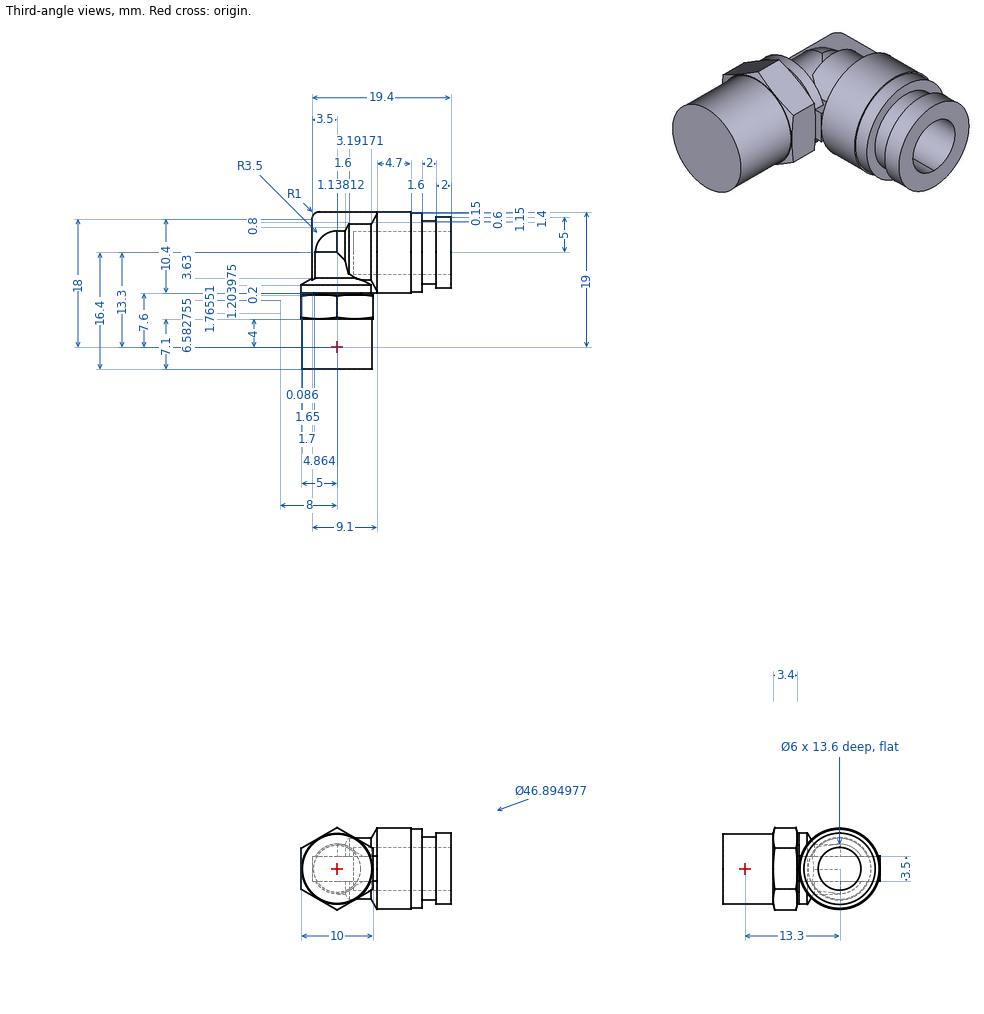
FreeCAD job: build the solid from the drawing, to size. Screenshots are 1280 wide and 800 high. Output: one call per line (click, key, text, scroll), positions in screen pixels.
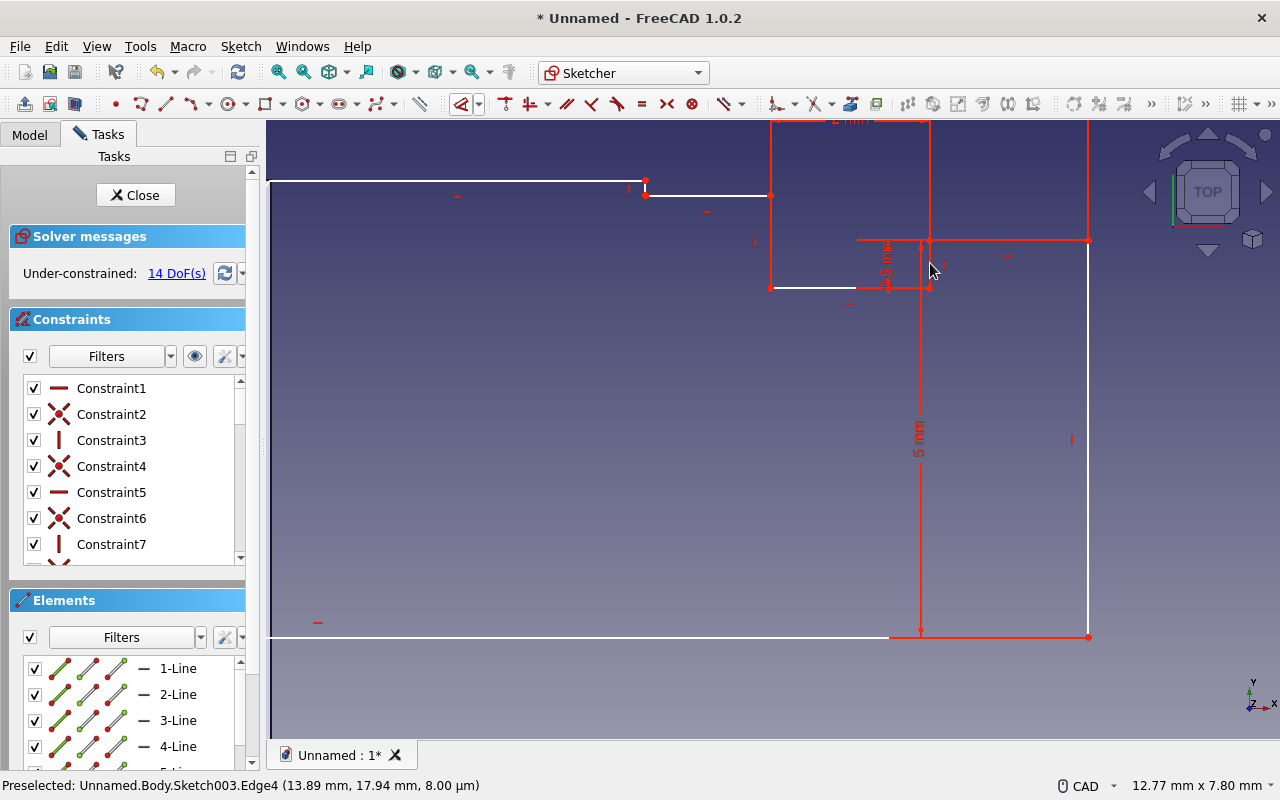
click(733, 196)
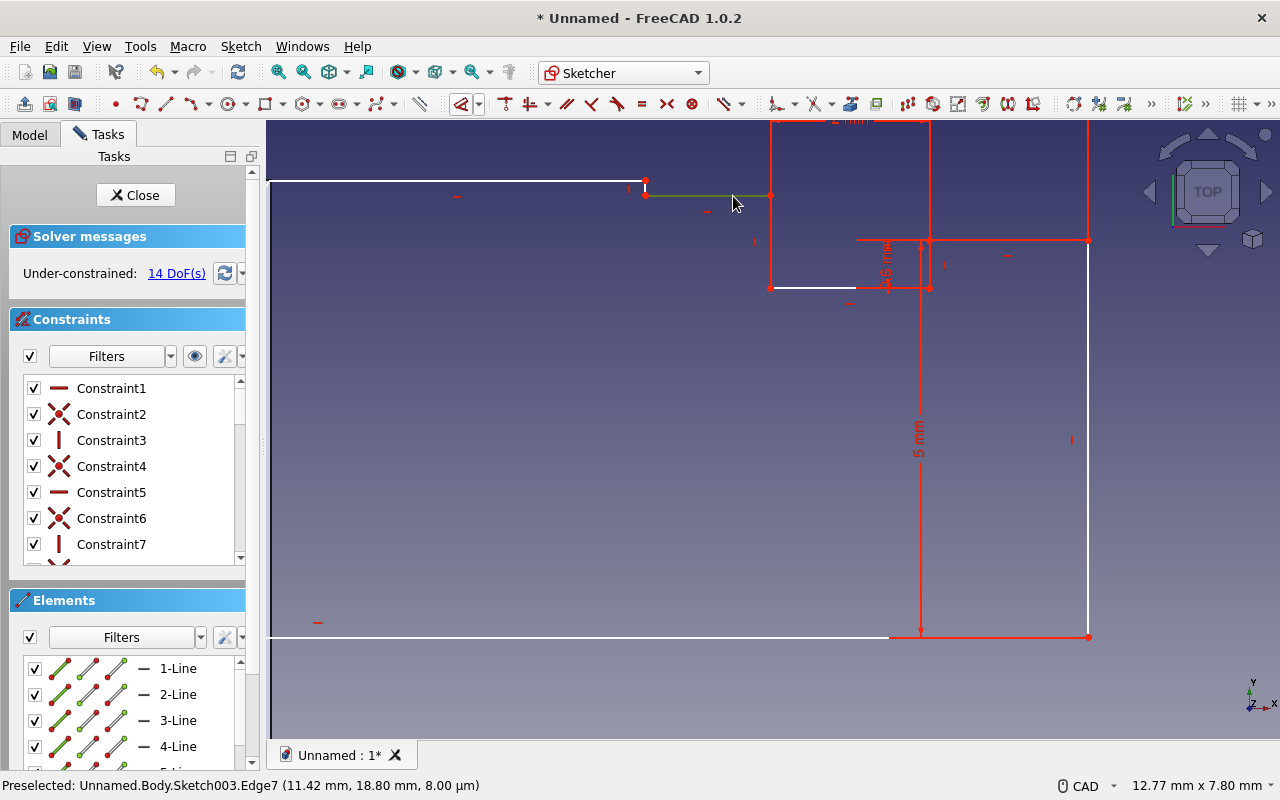
key(l)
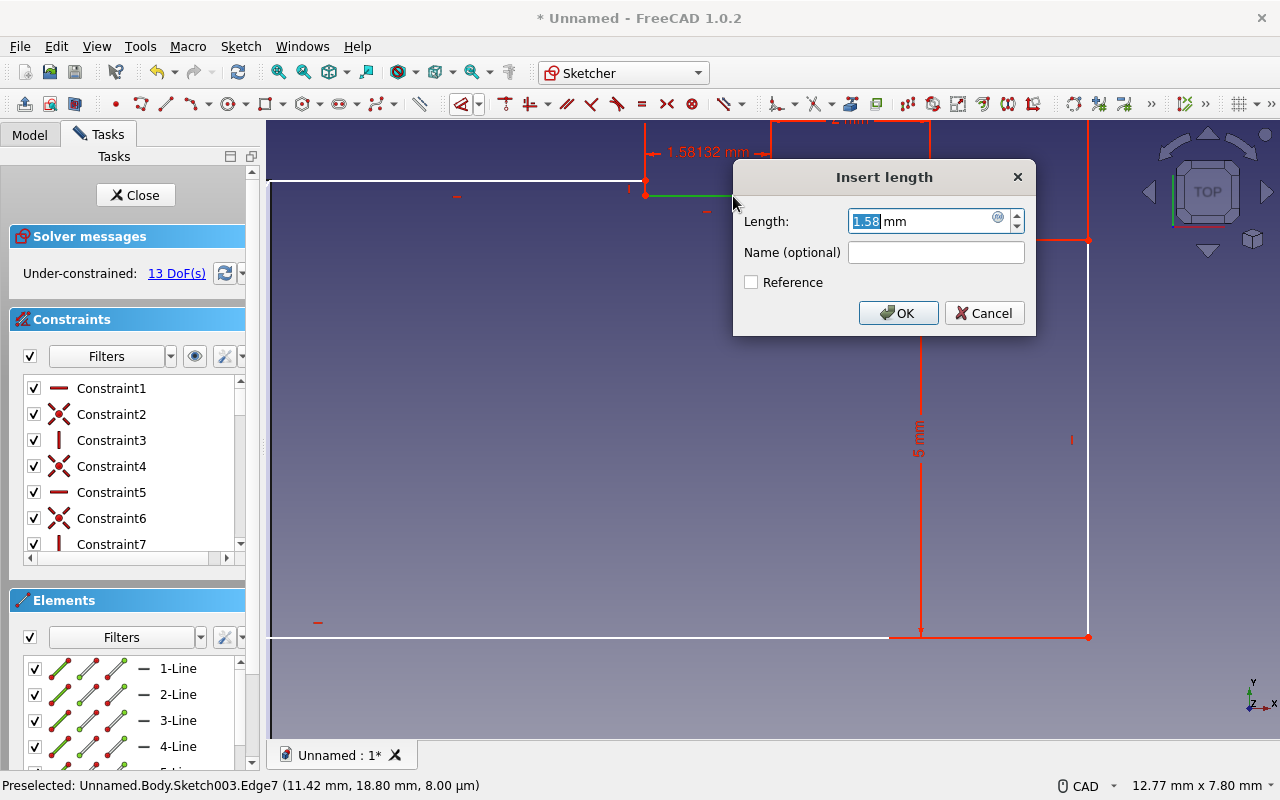
text(1.6)
key(Return)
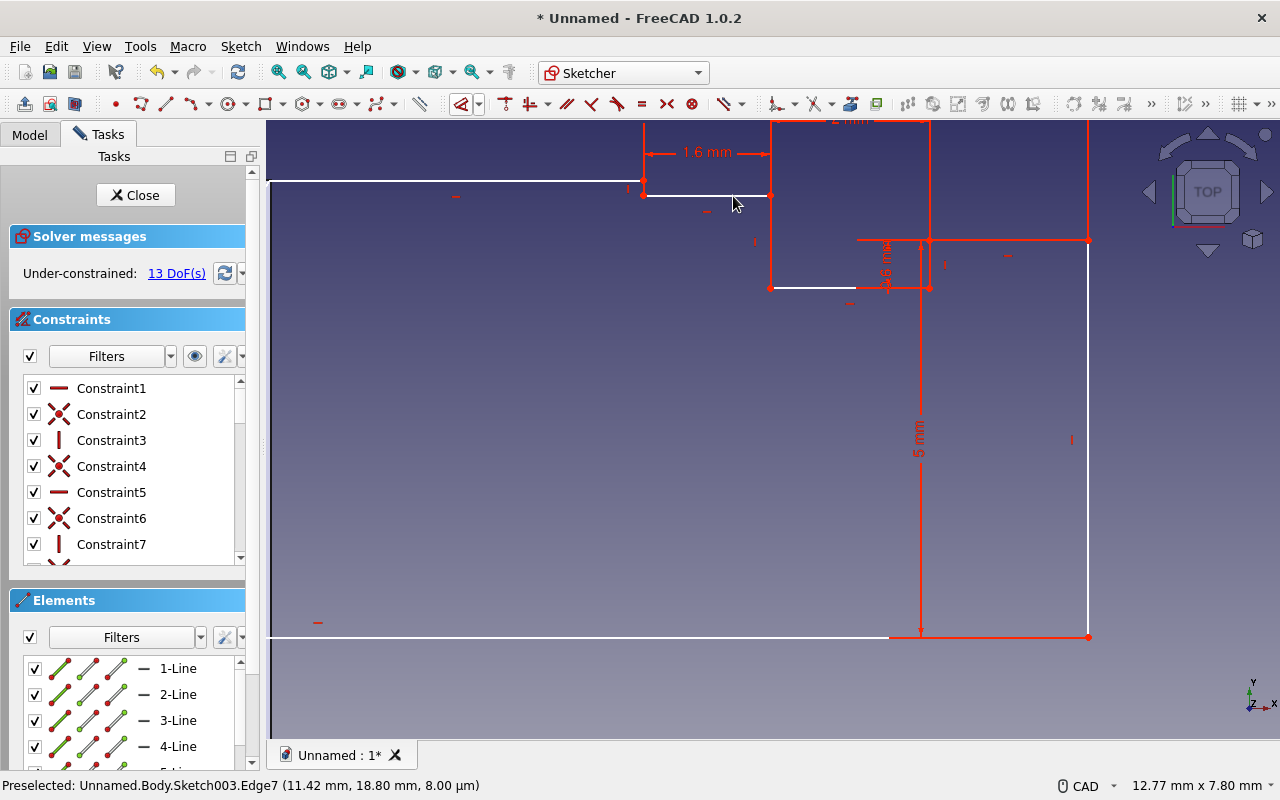
scroll(932, 264, down, 7)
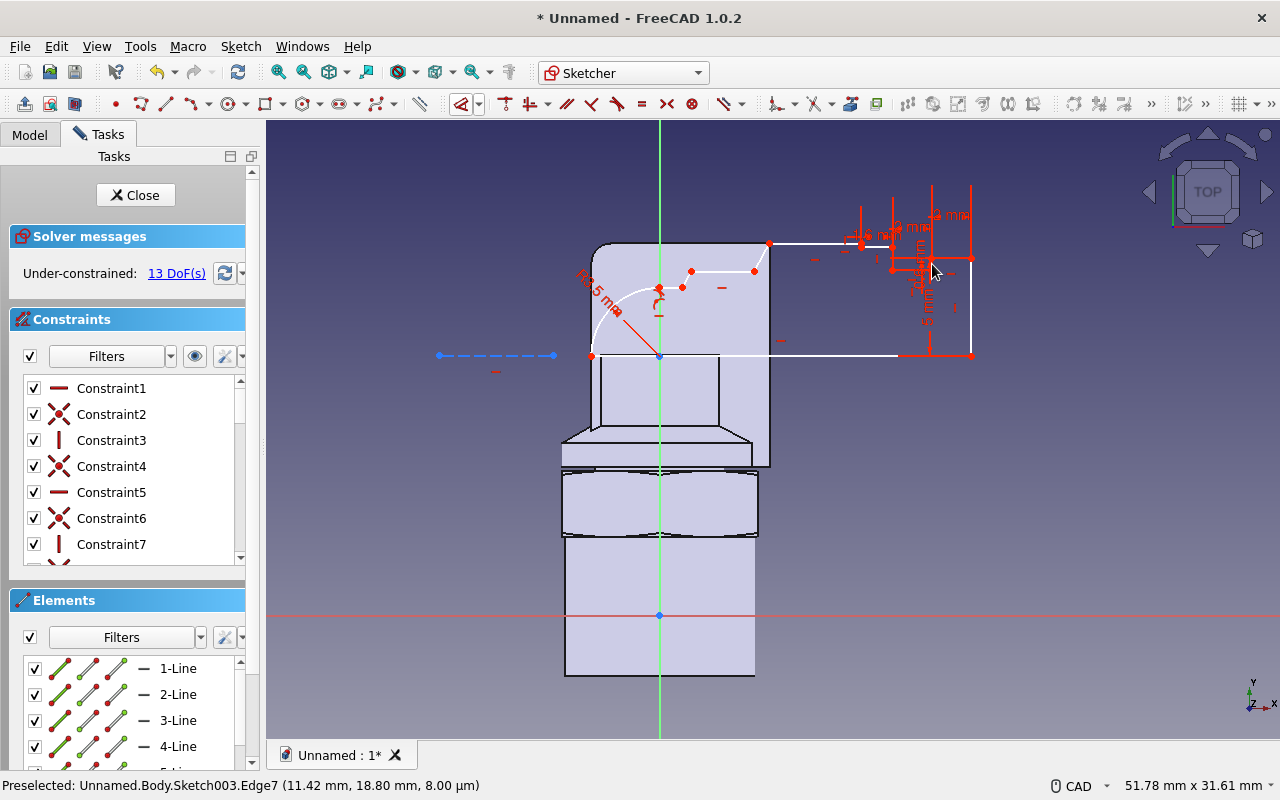
click(834, 244)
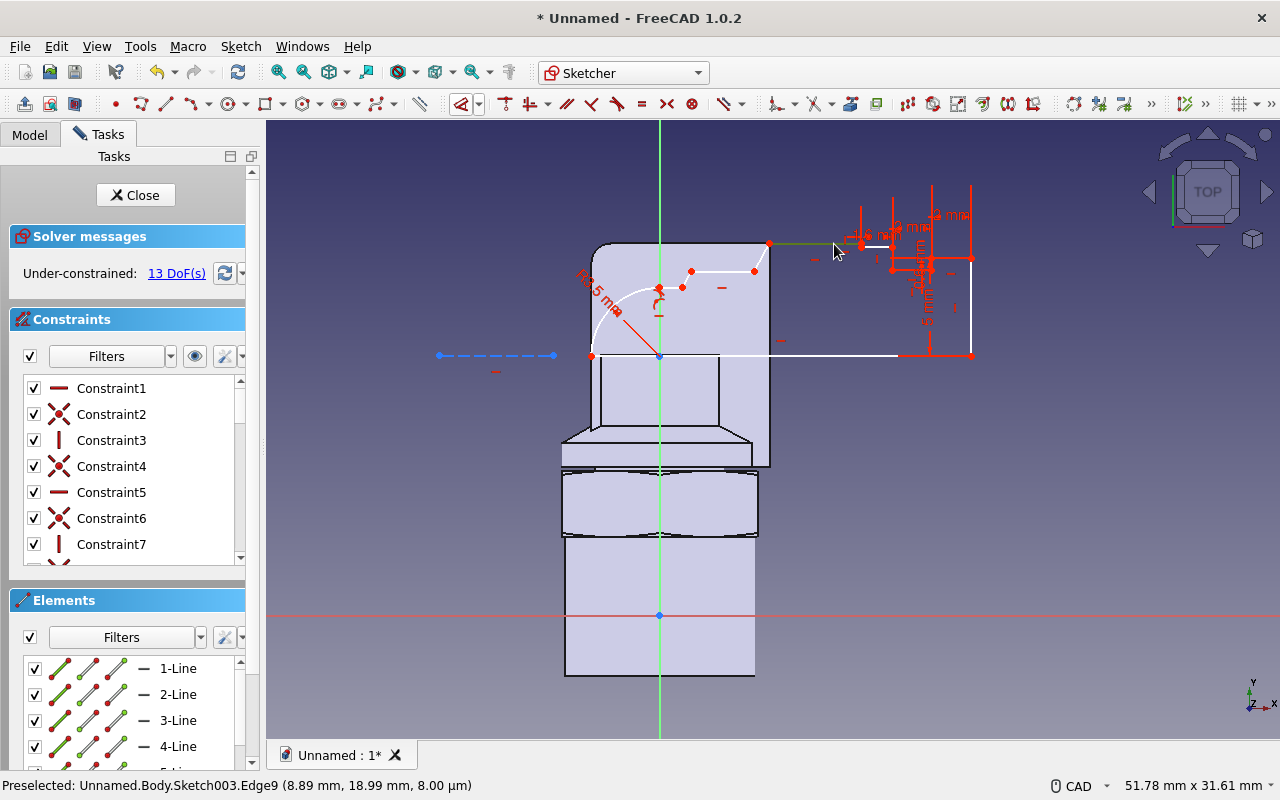
key(l)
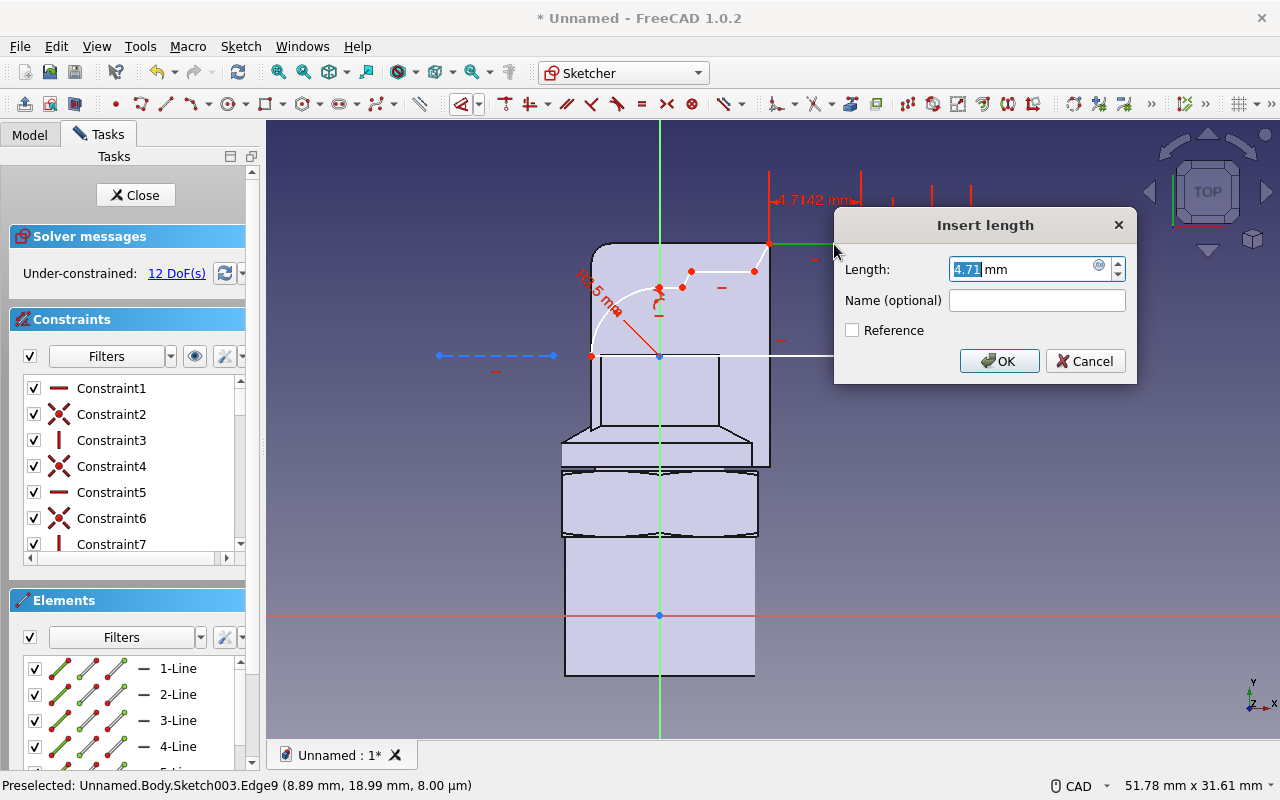
text(4.7)
key(Return)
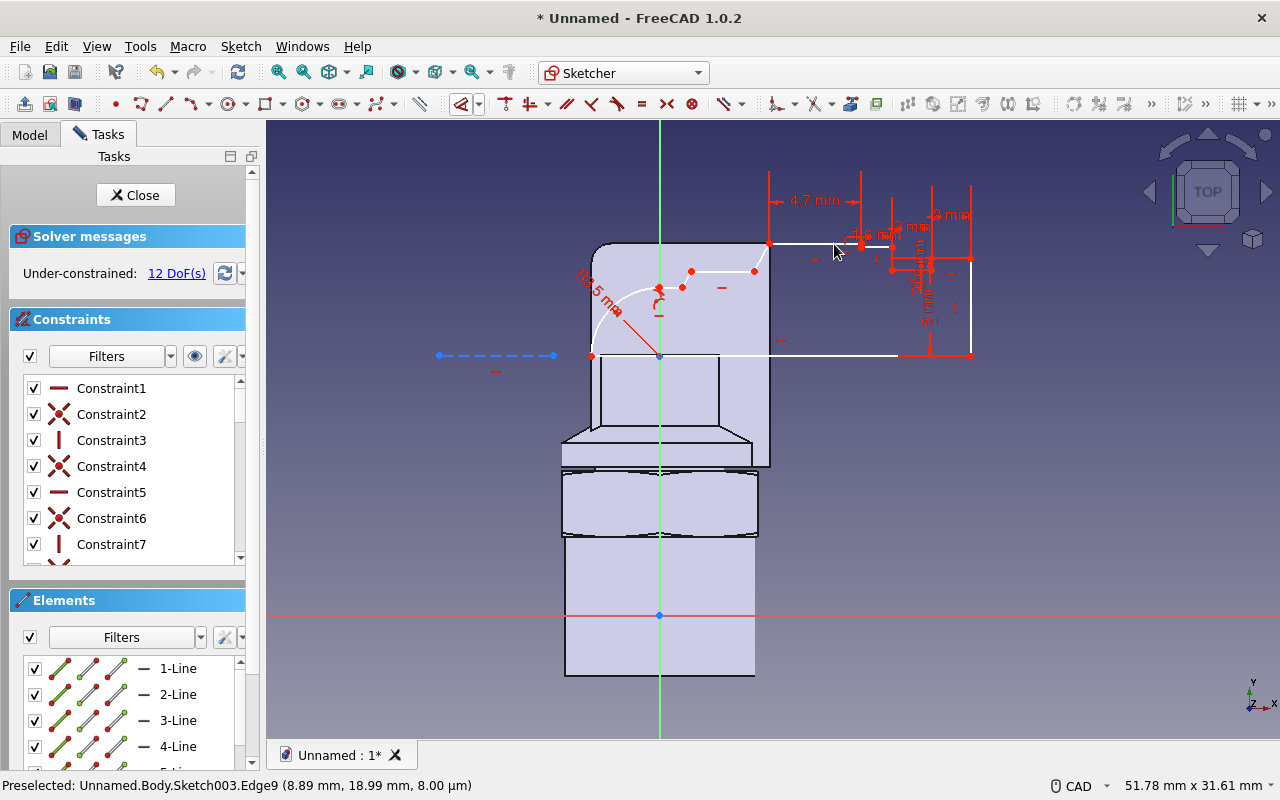
scroll(861, 244, up, 7)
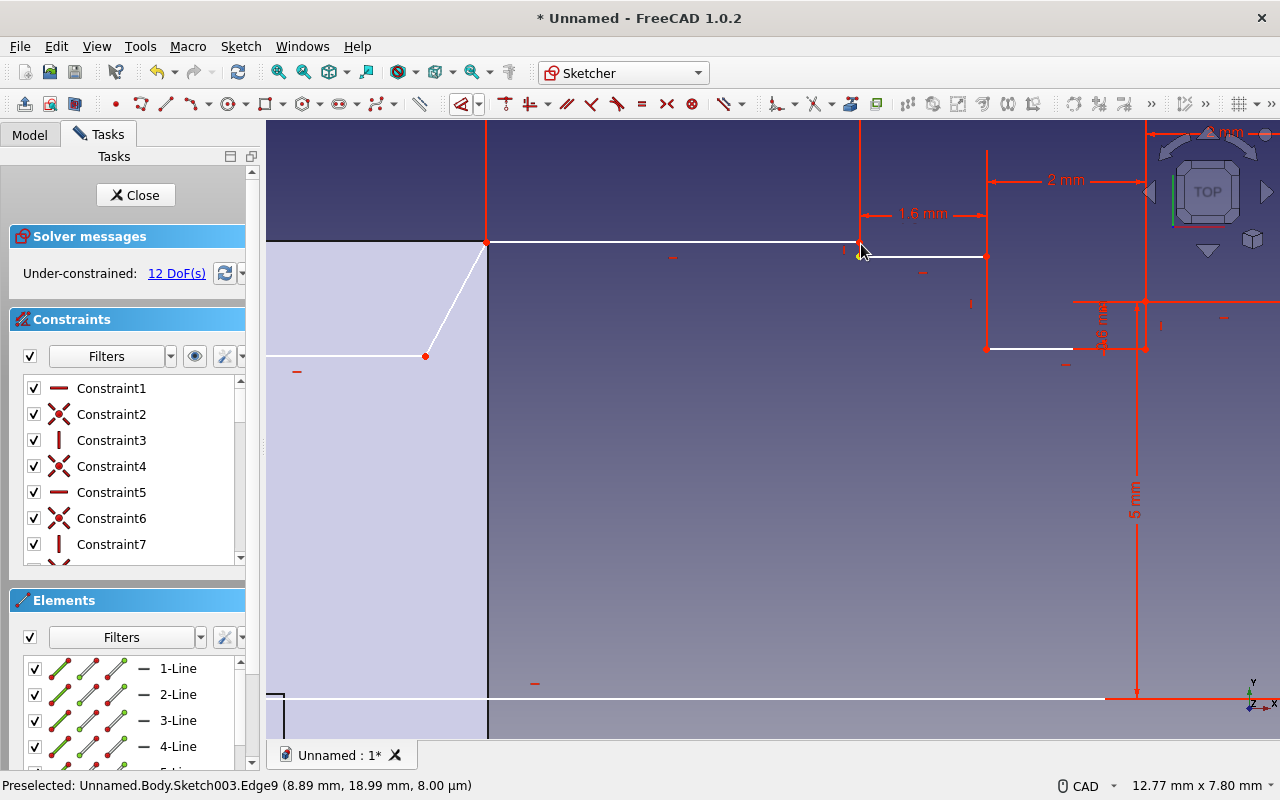
click(860, 242)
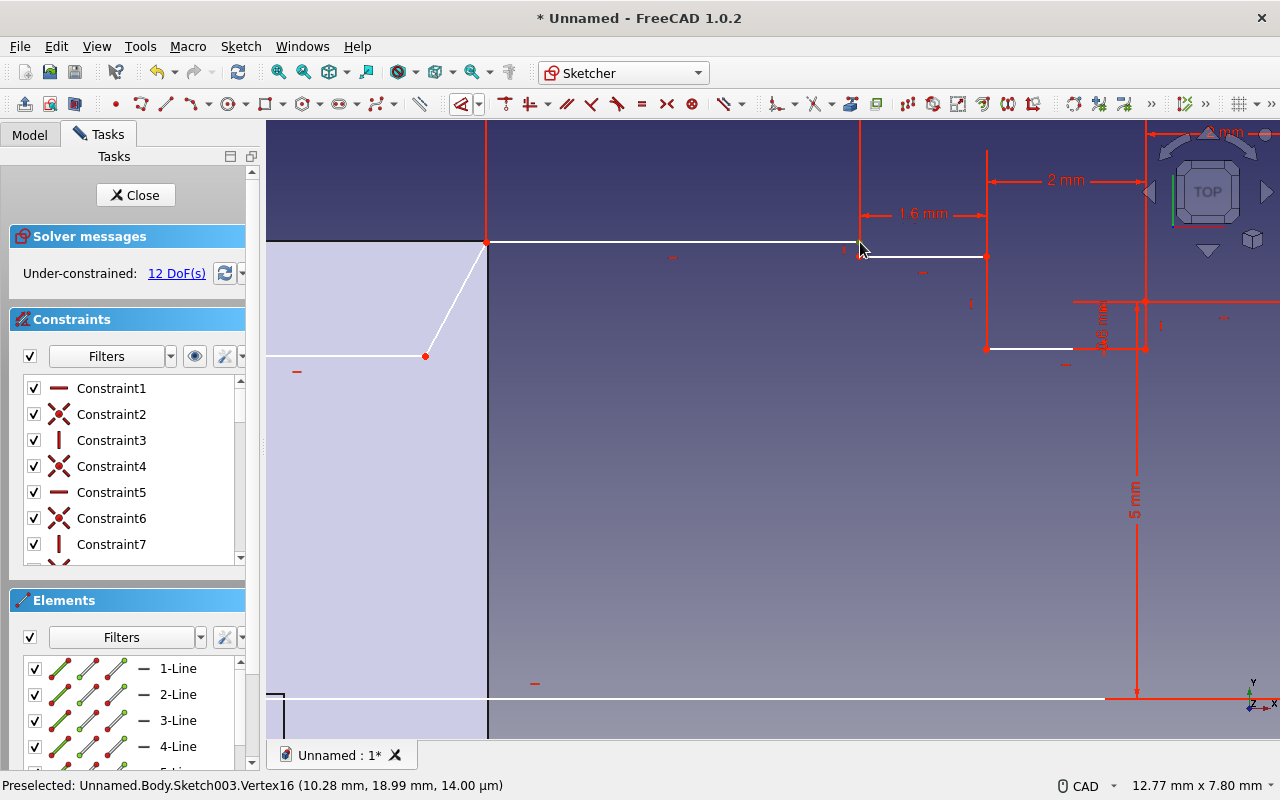
click(478, 104)